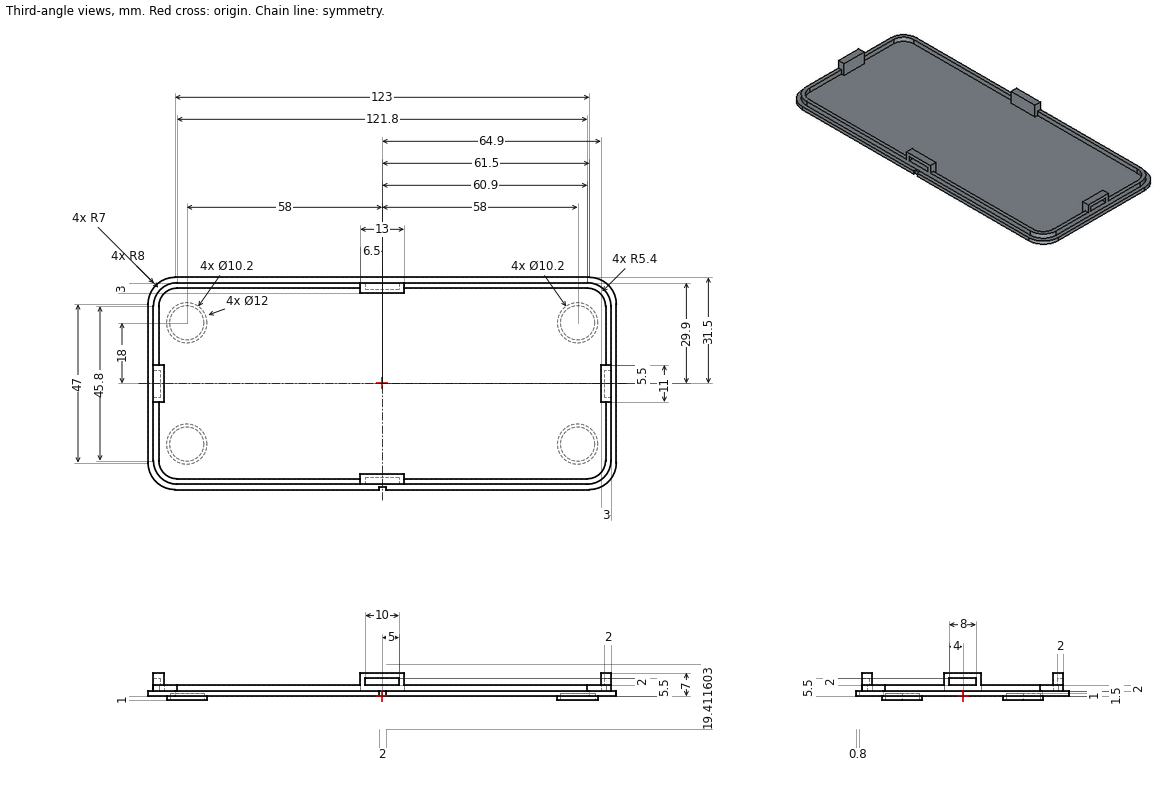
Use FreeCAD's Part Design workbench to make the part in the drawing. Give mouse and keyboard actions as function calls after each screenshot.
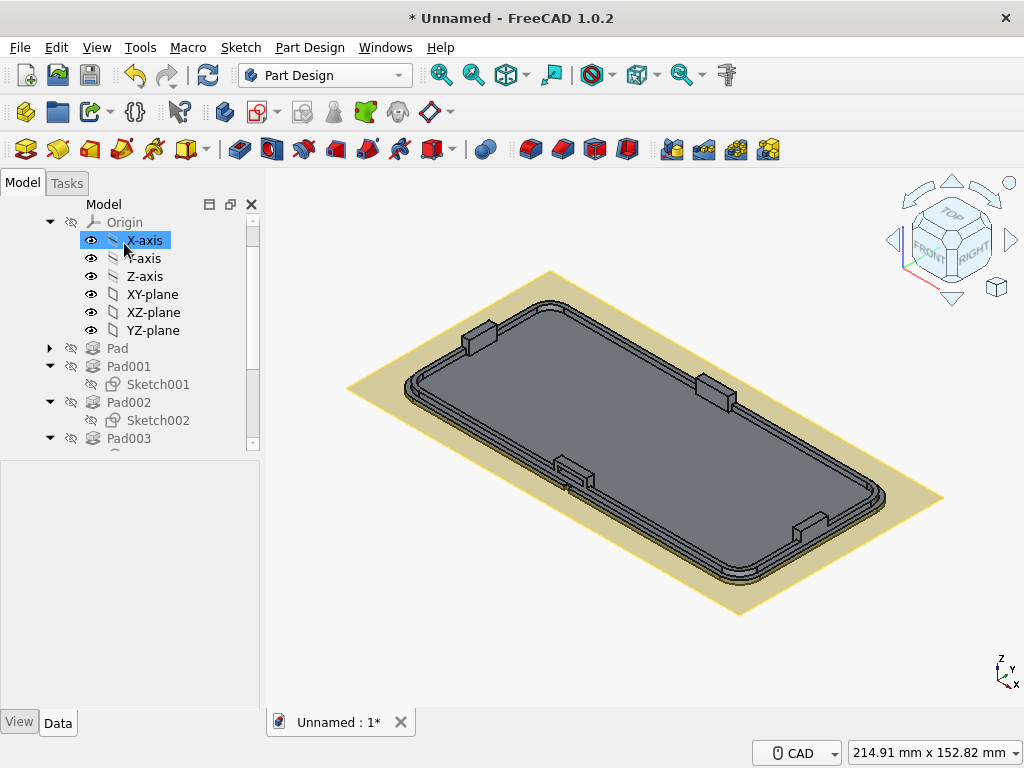
scroll(140, 326, down, 3)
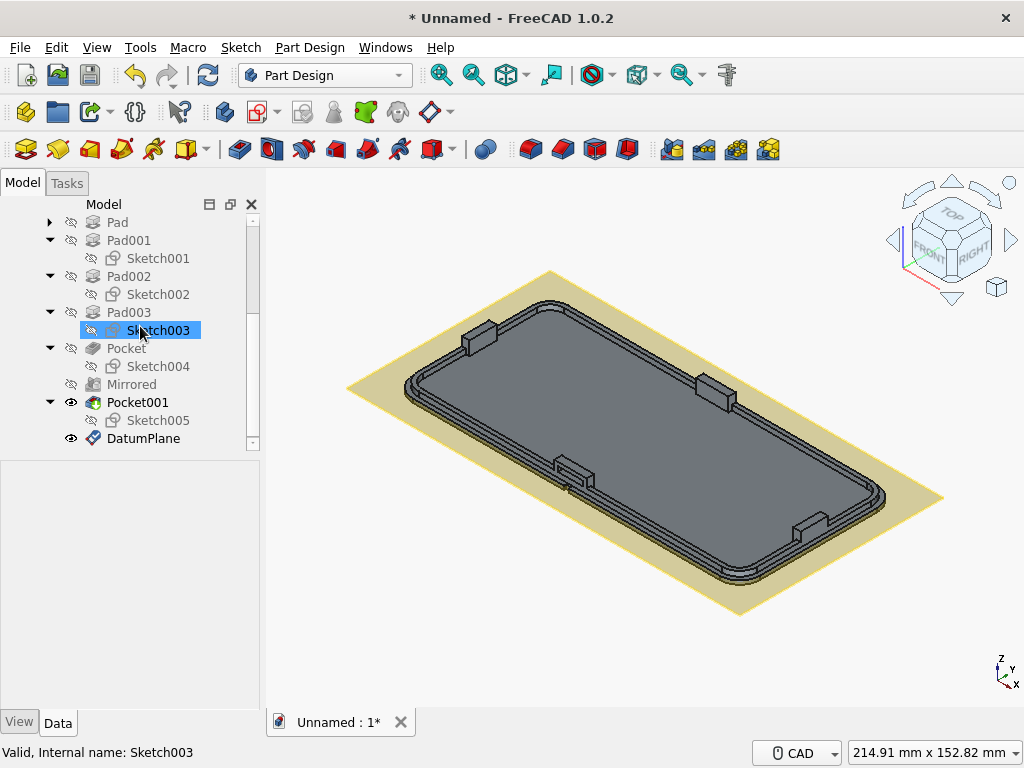
click(116, 438)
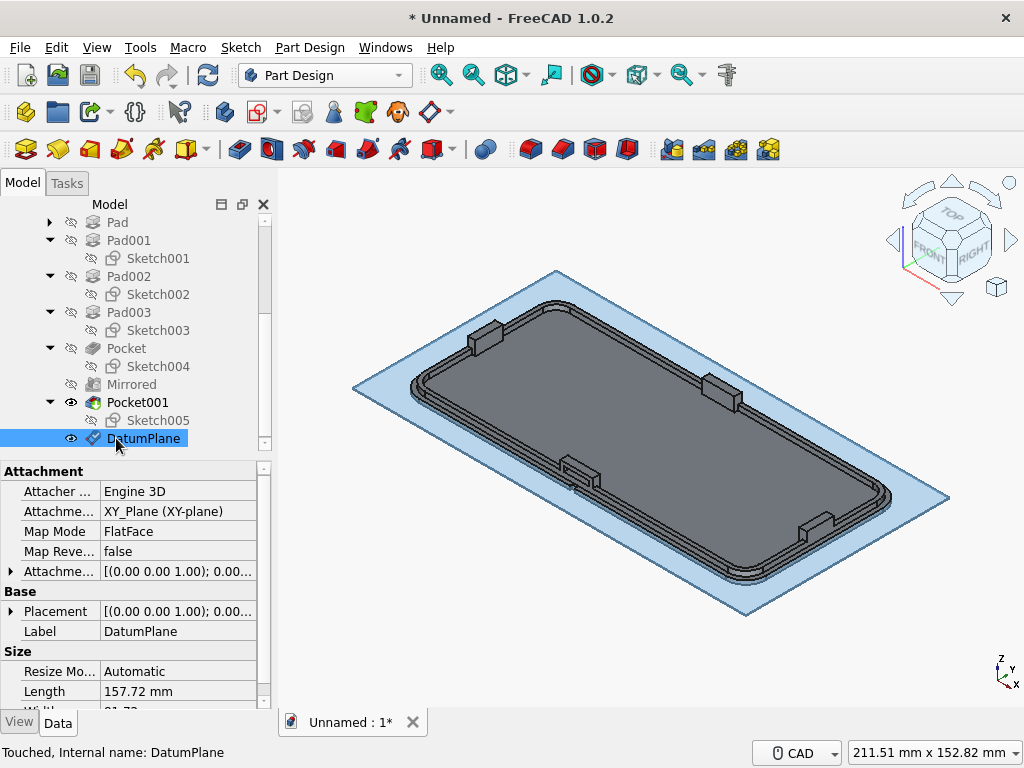
click(258, 112)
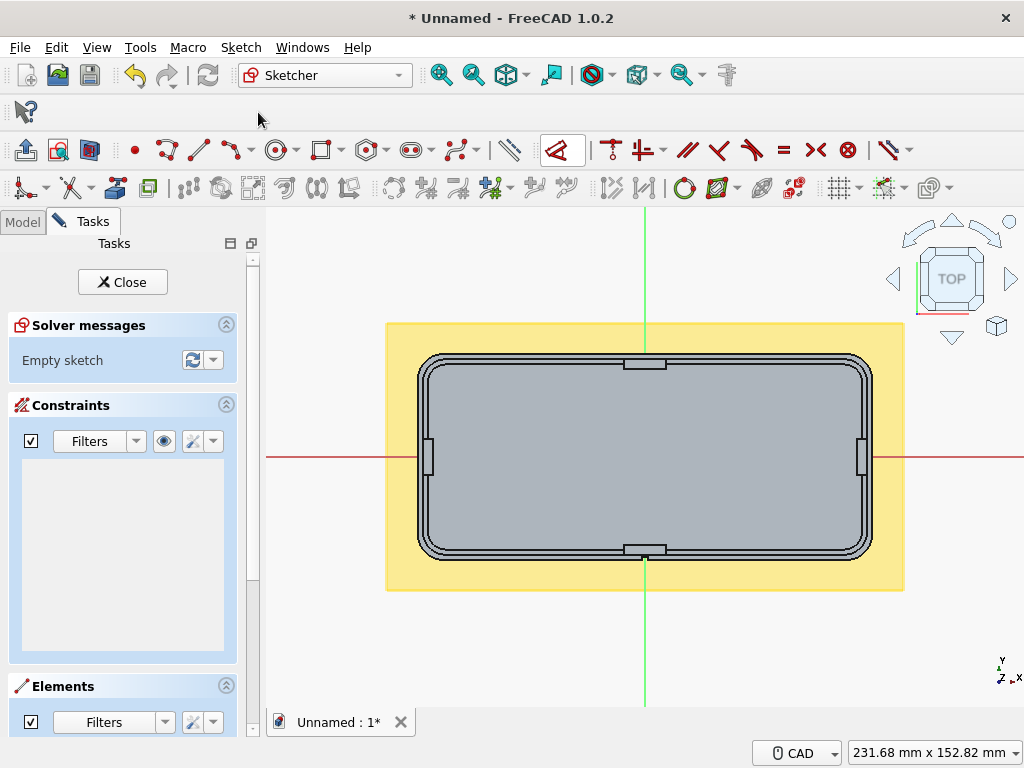
key(q)
key(s)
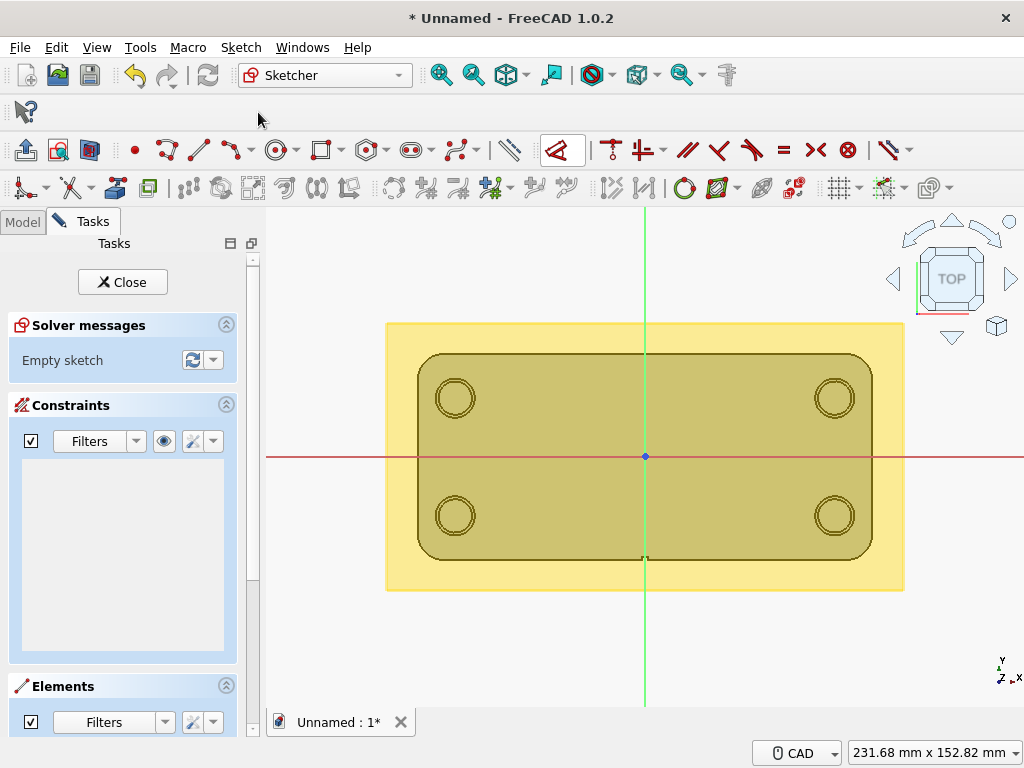
scroll(294, 457, down, 1)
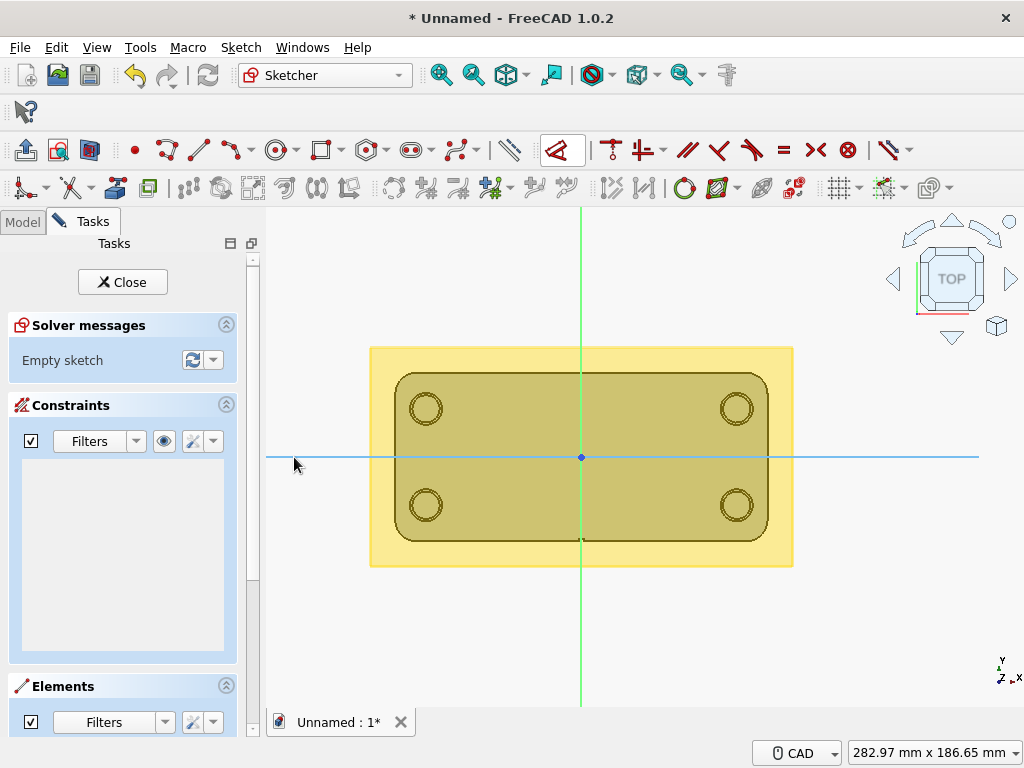
click(276, 150)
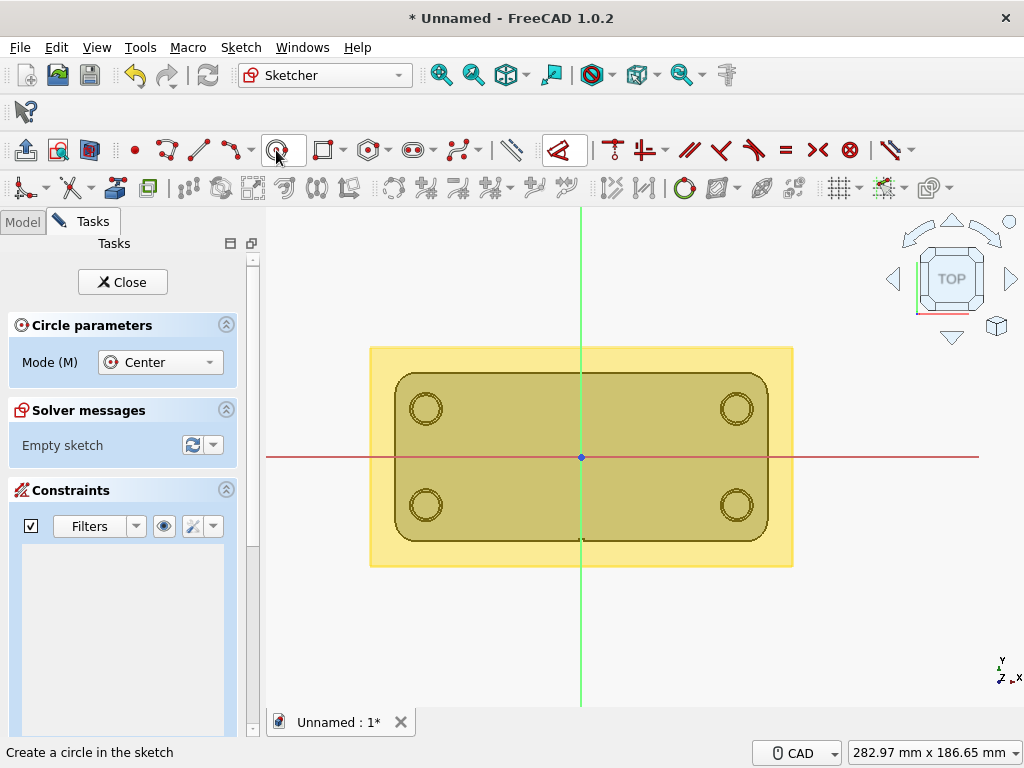
scroll(737, 409, up, 3)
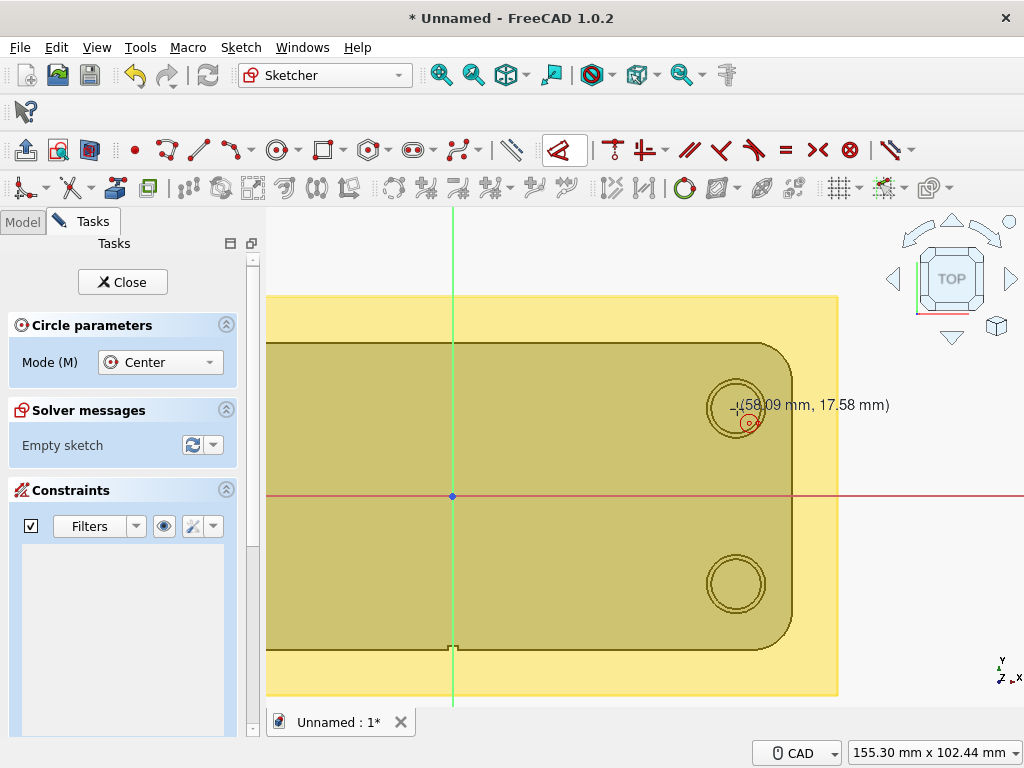
click(736, 408)
click(754, 391)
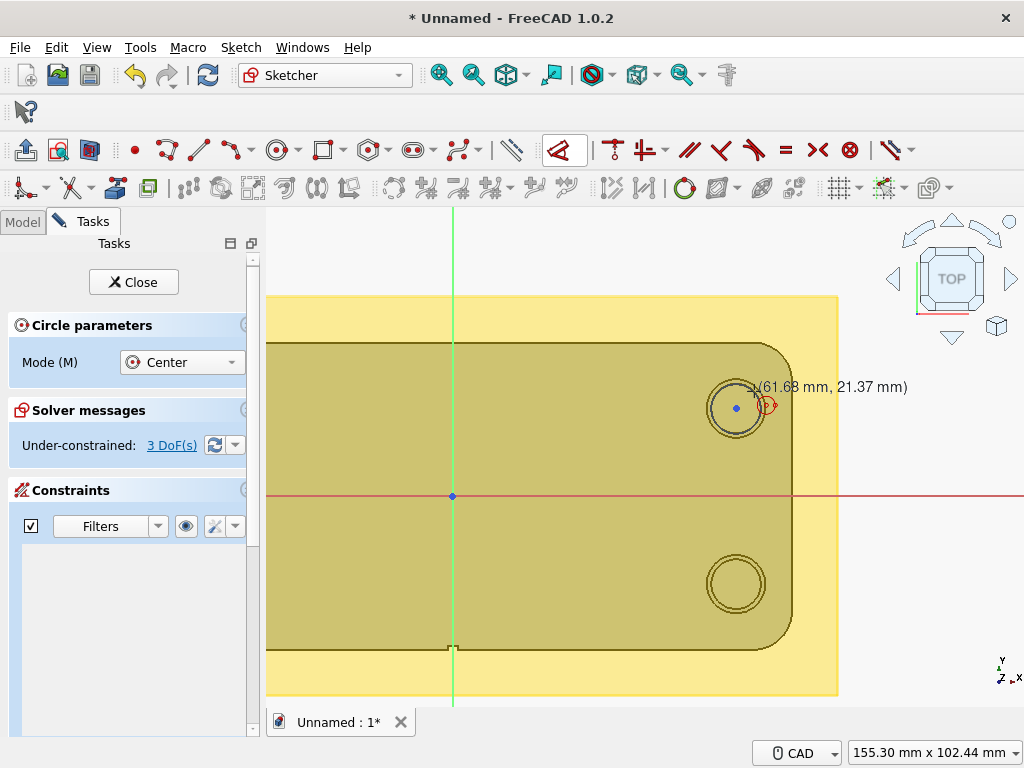
scroll(828, 377, down, 2)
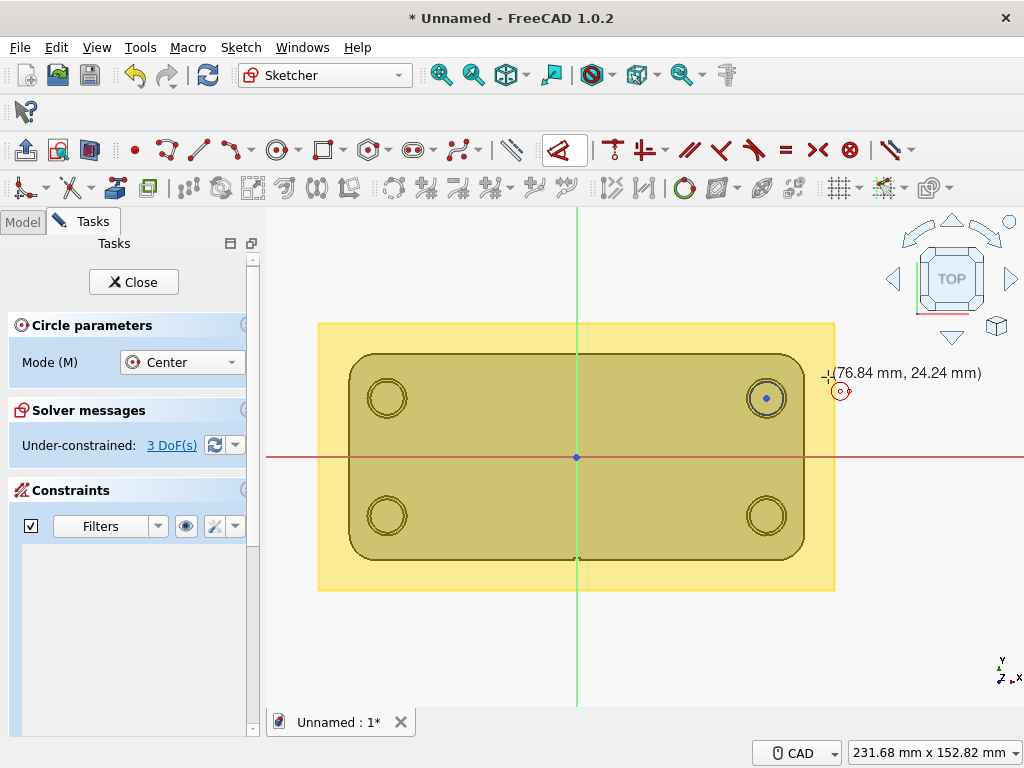
scroll(387, 398, up, 2)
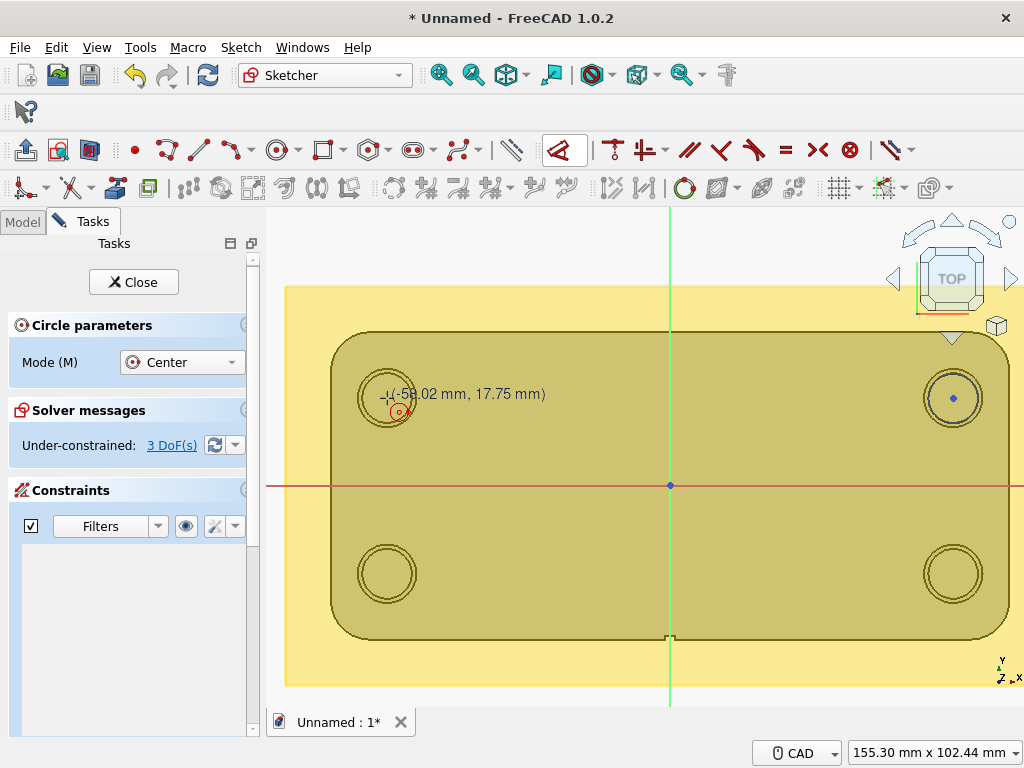
click(387, 398)
click(405, 380)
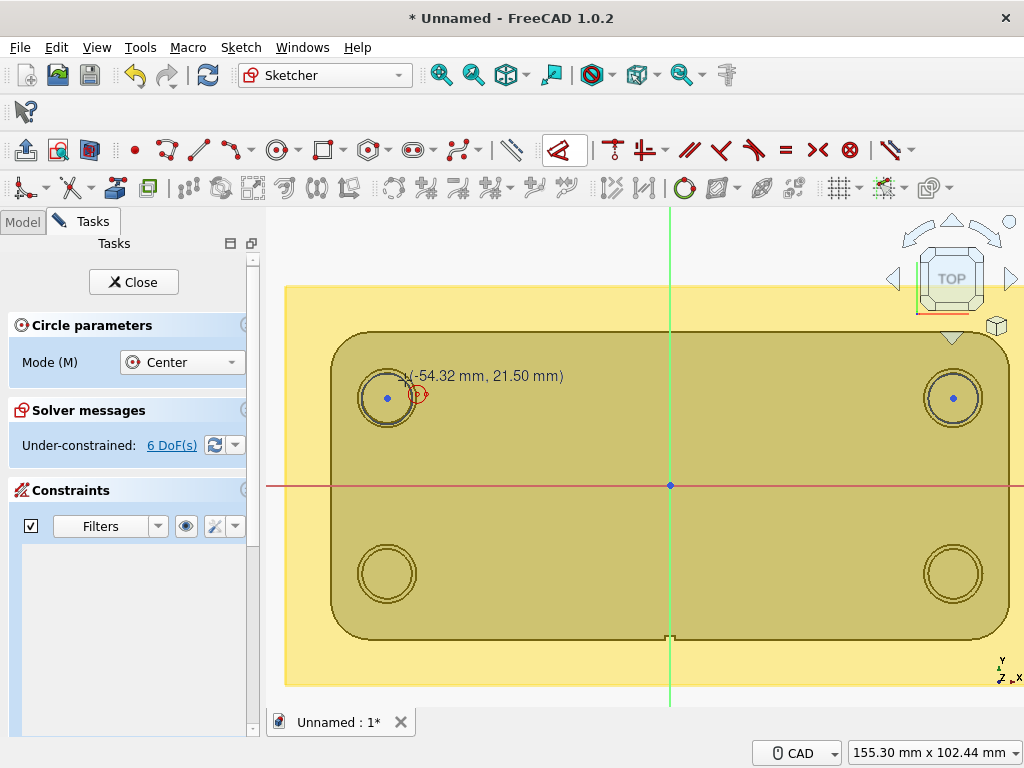
click(387, 574)
click(405, 556)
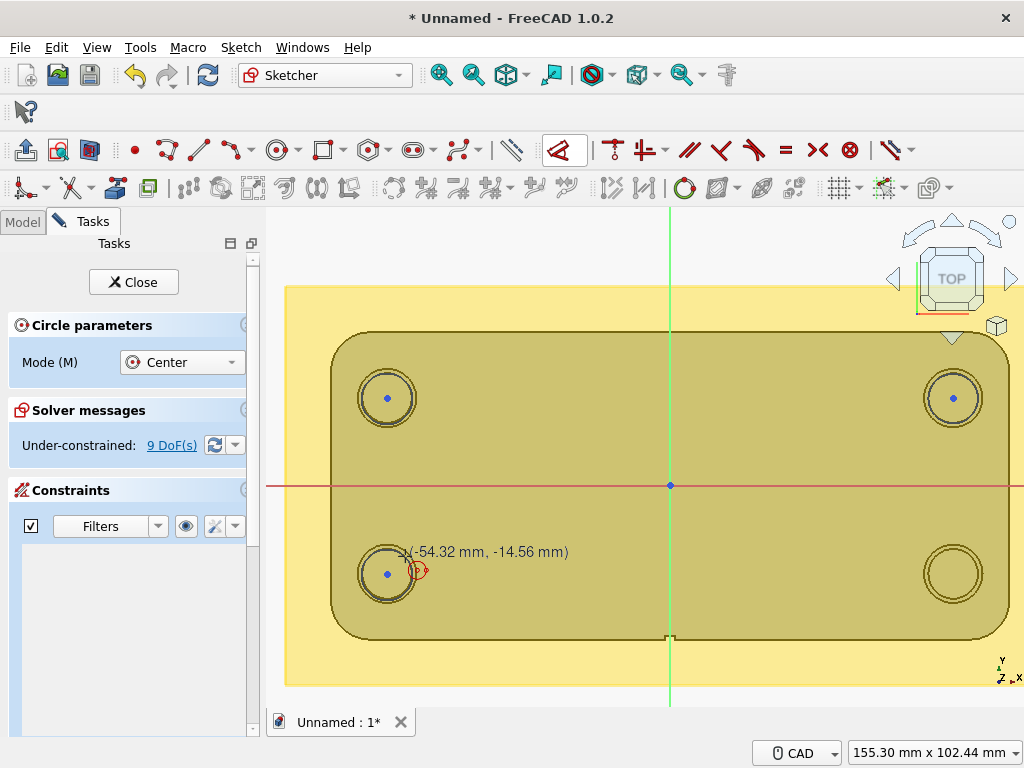
scroll(386, 398, down, 2)